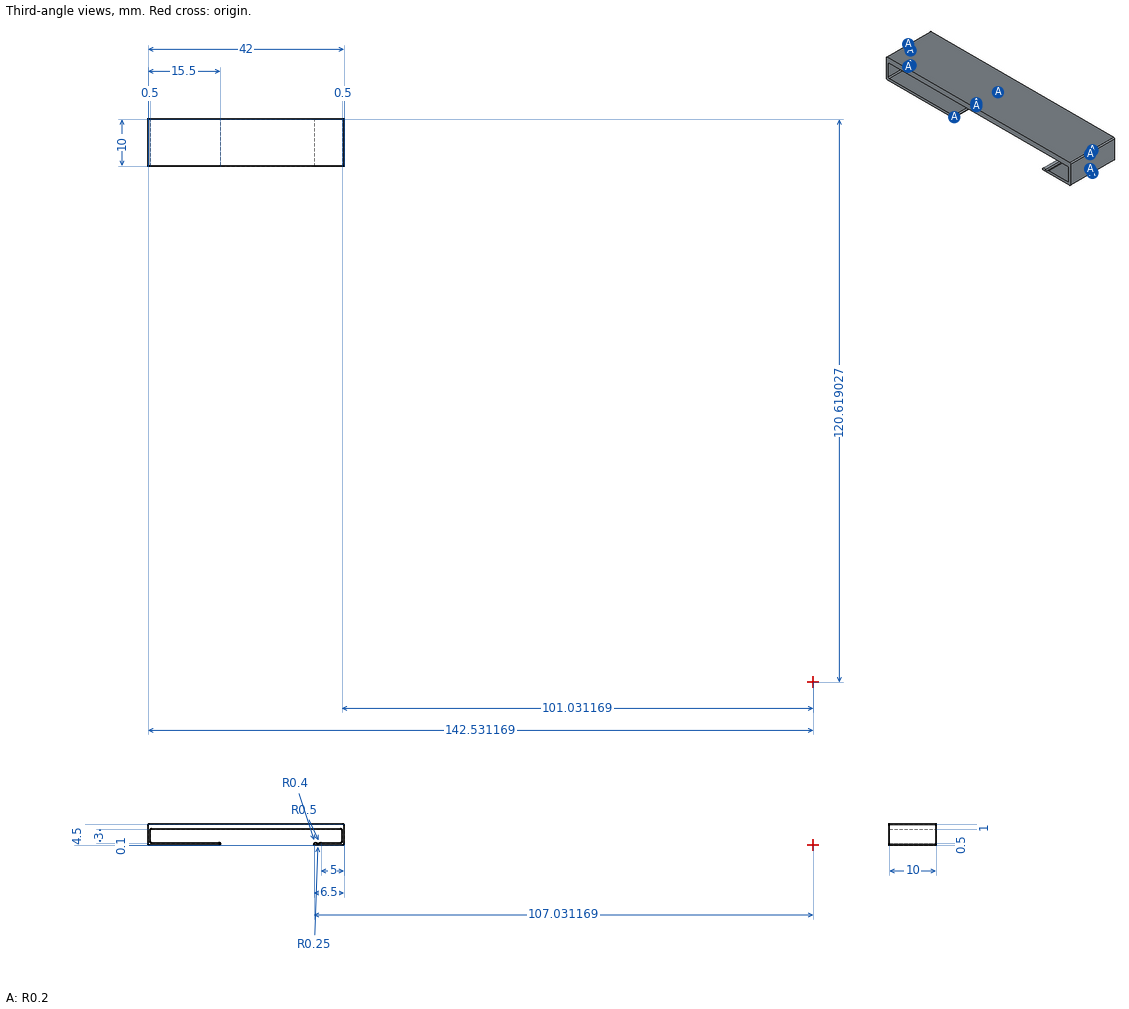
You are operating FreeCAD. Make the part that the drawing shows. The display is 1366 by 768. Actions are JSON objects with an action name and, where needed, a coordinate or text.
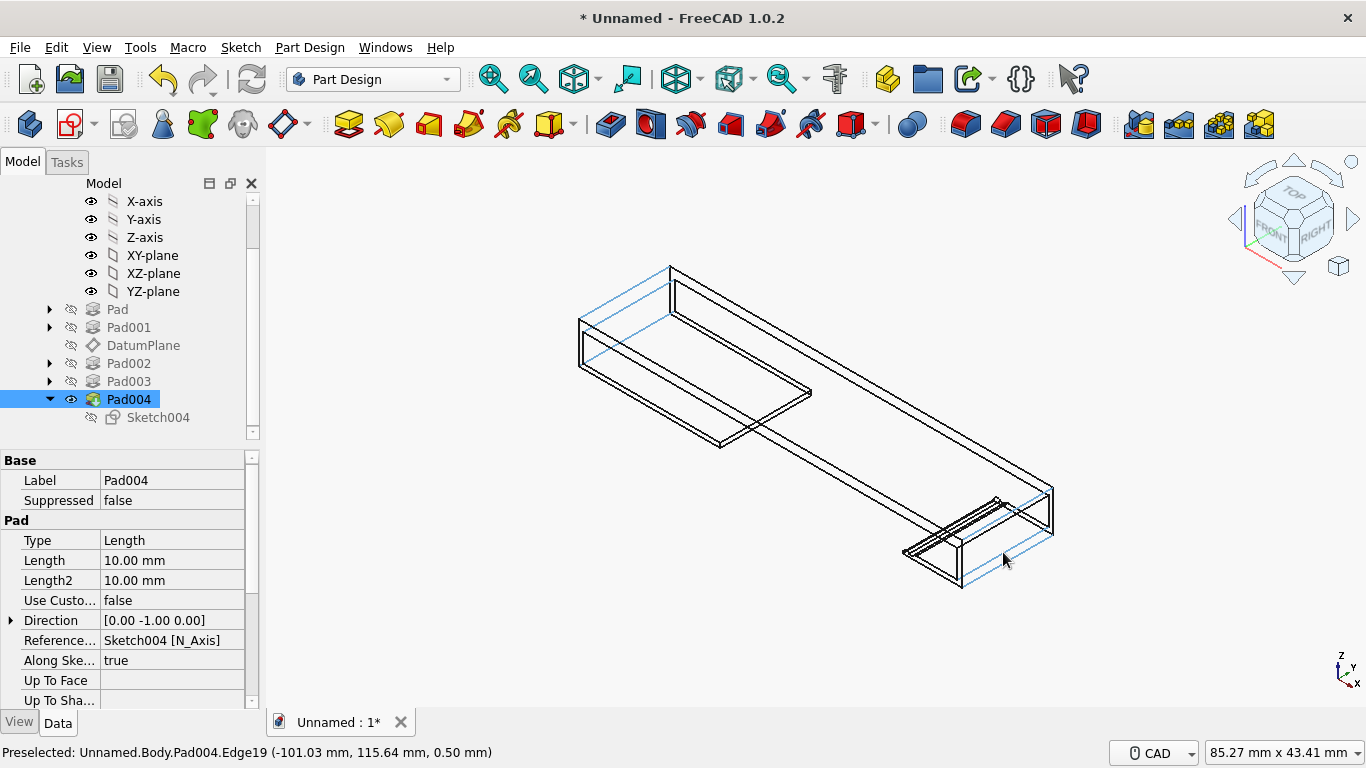
{"action": "scroll", "coordinate": [1003, 521], "scroll_direction": "up", "scroll_amount": 6}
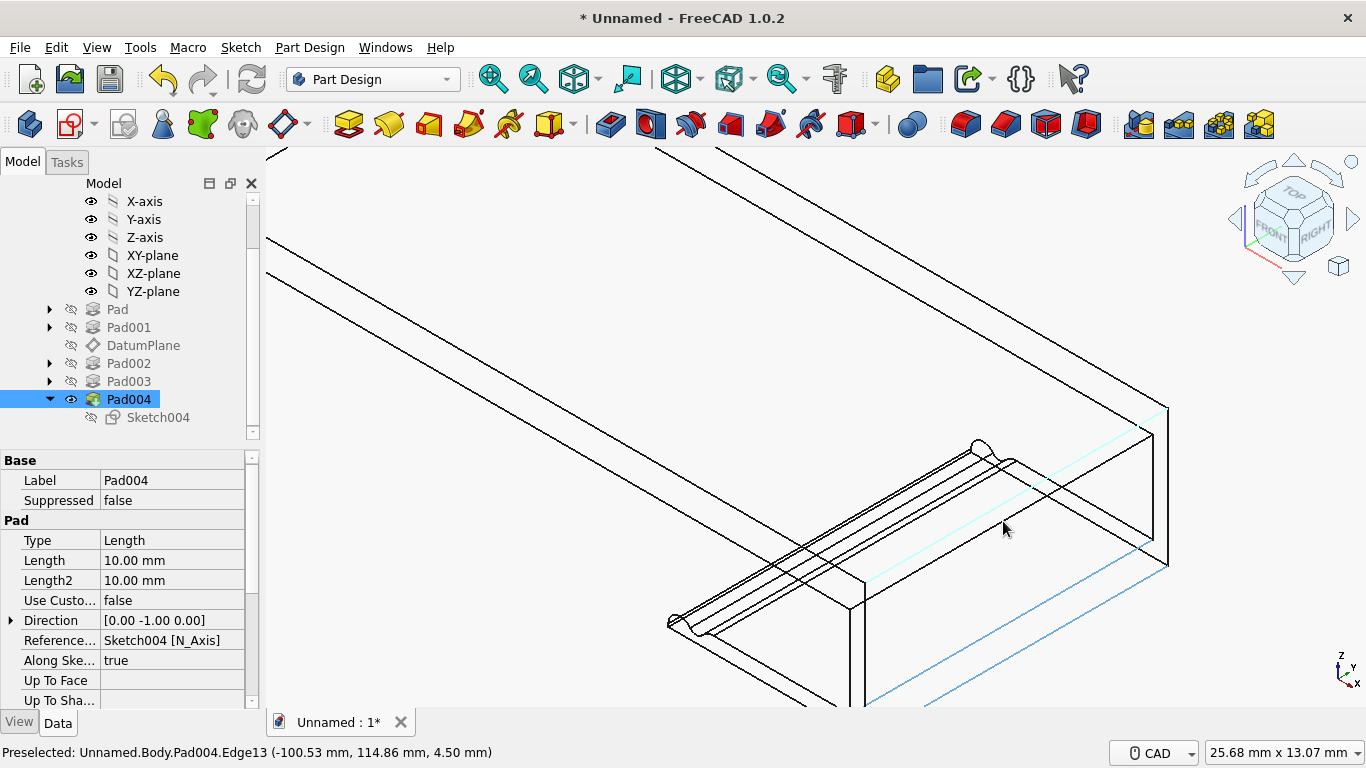
{"action": "left_click", "coordinate": [1001, 521], "text": "ctrl"}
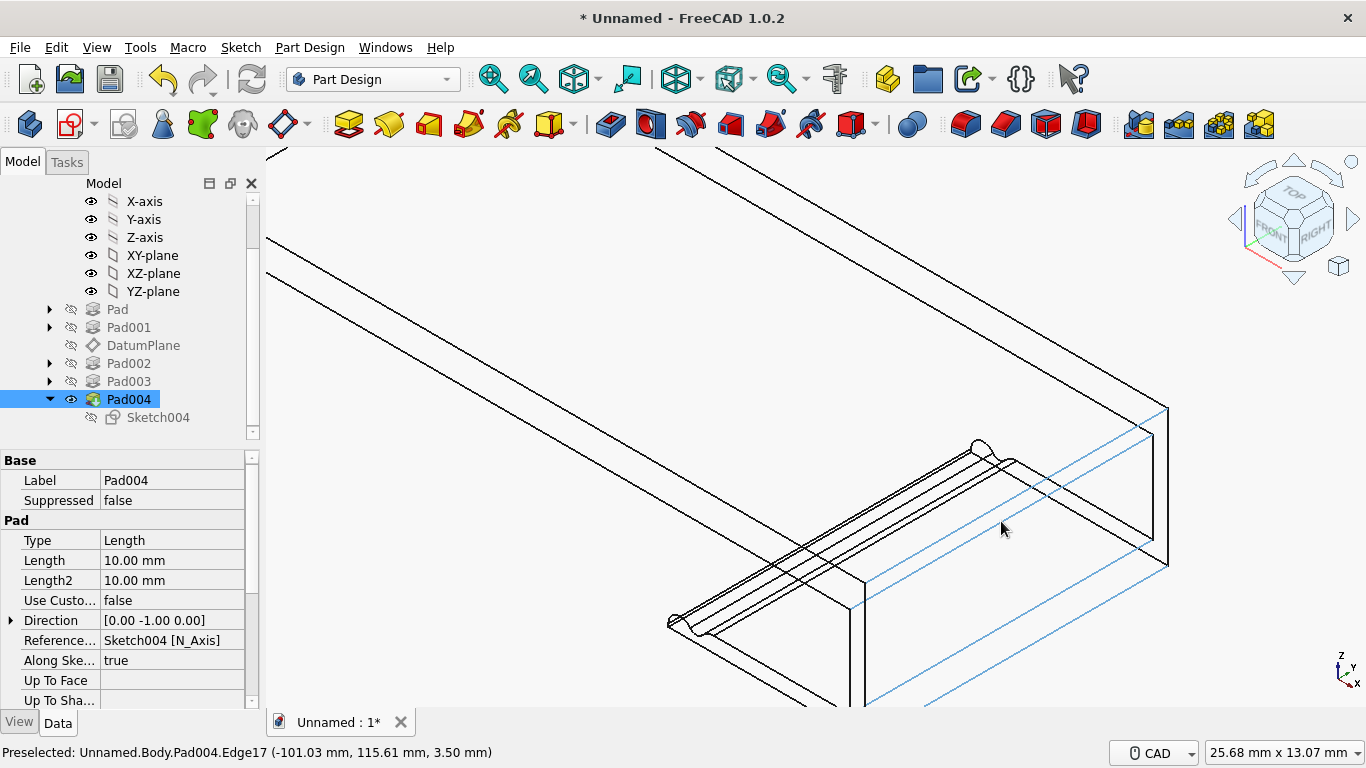
{"action": "key", "text": "v 1"}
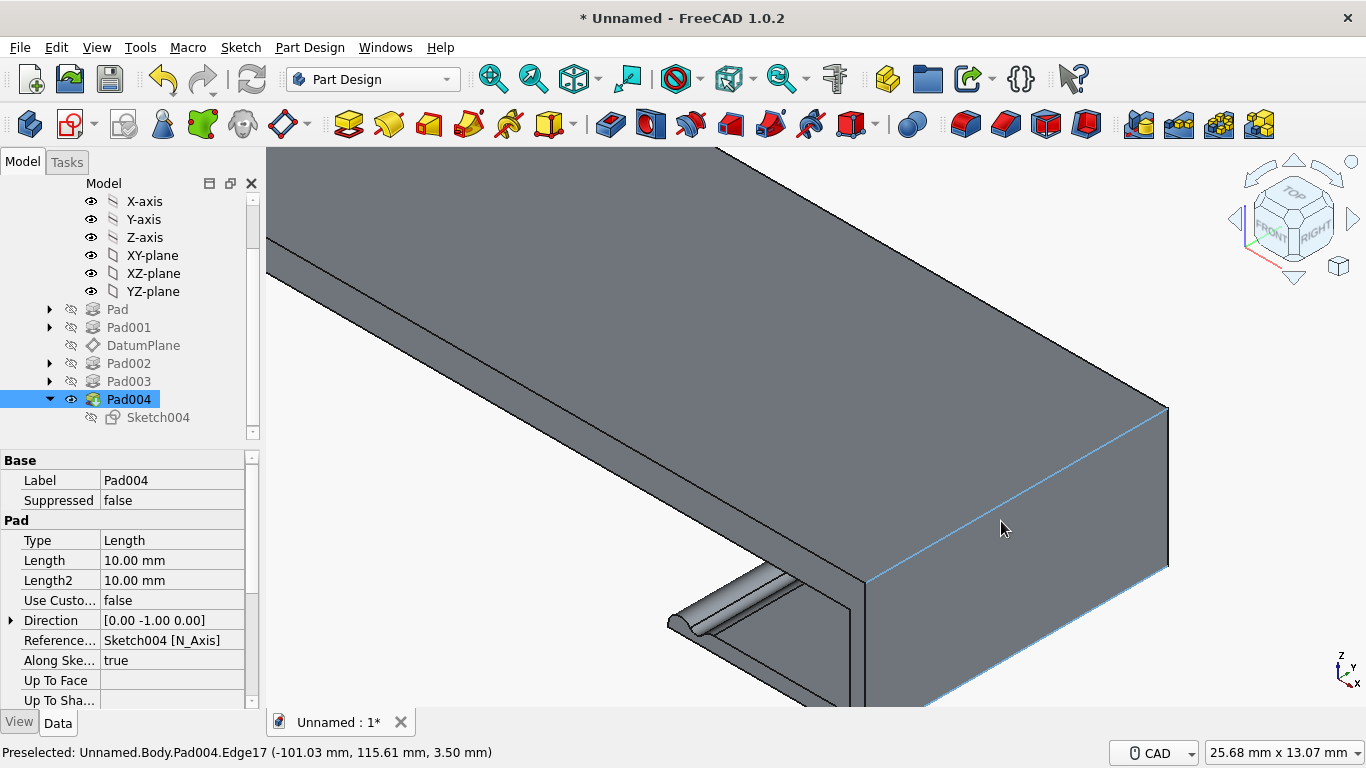
{"action": "left_click", "coordinate": [966, 124]}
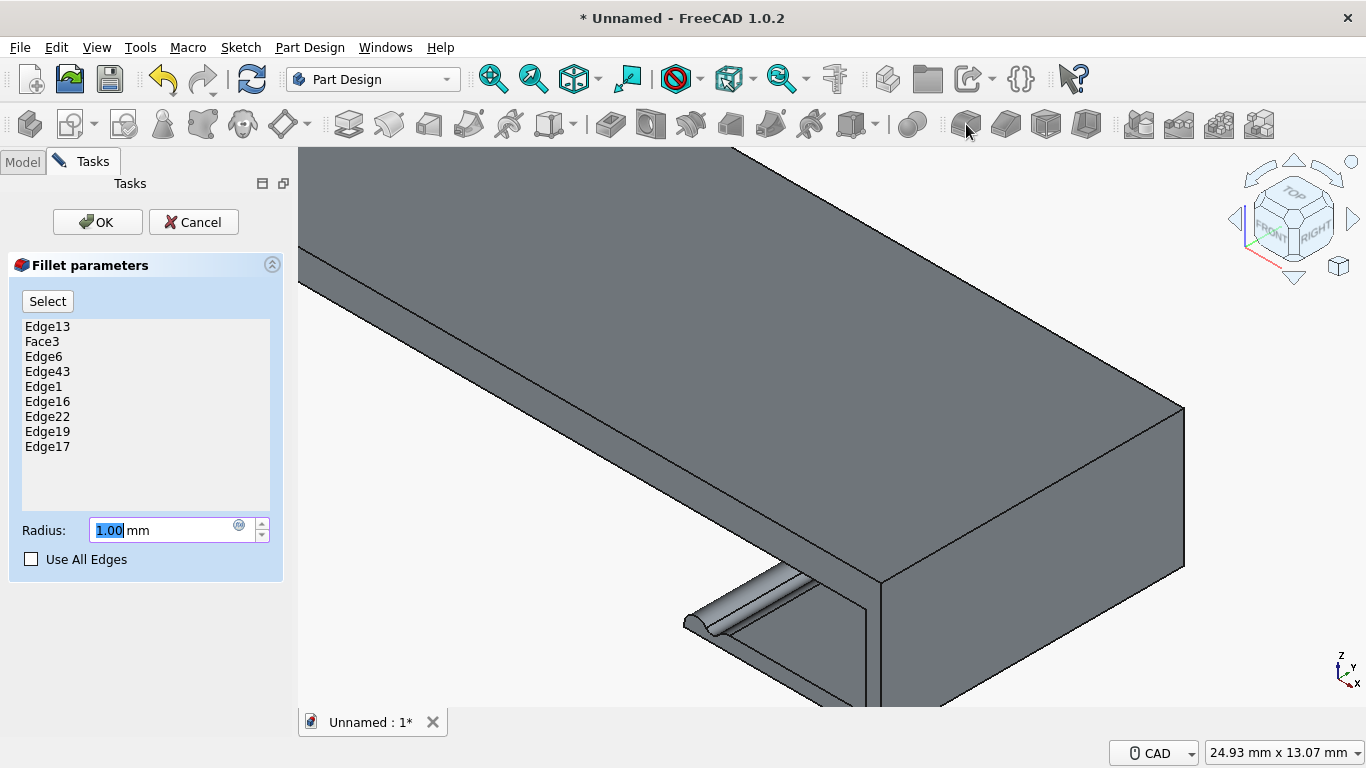
{"action": "type", "text": "0.2"}
{"action": "key", "text": "Tab"}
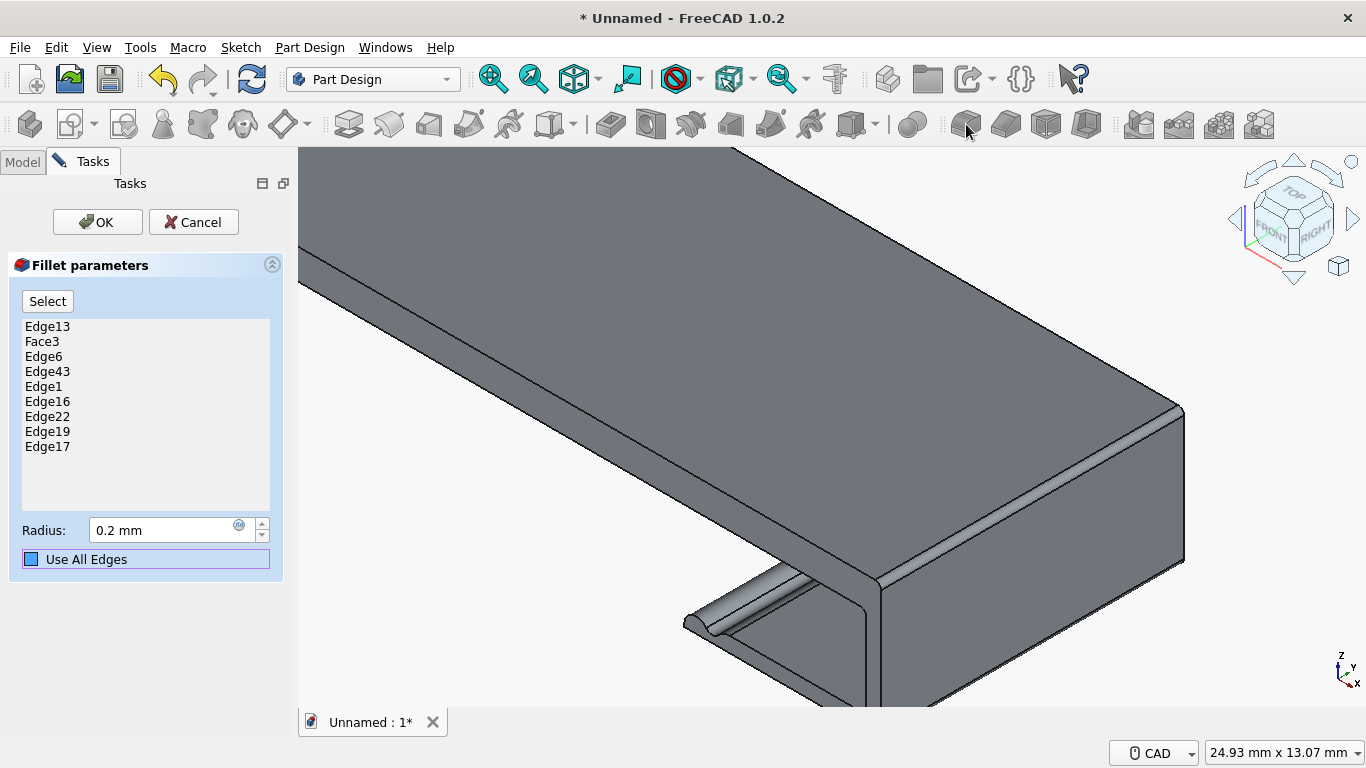
{"action": "left_click", "coordinate": [98, 222]}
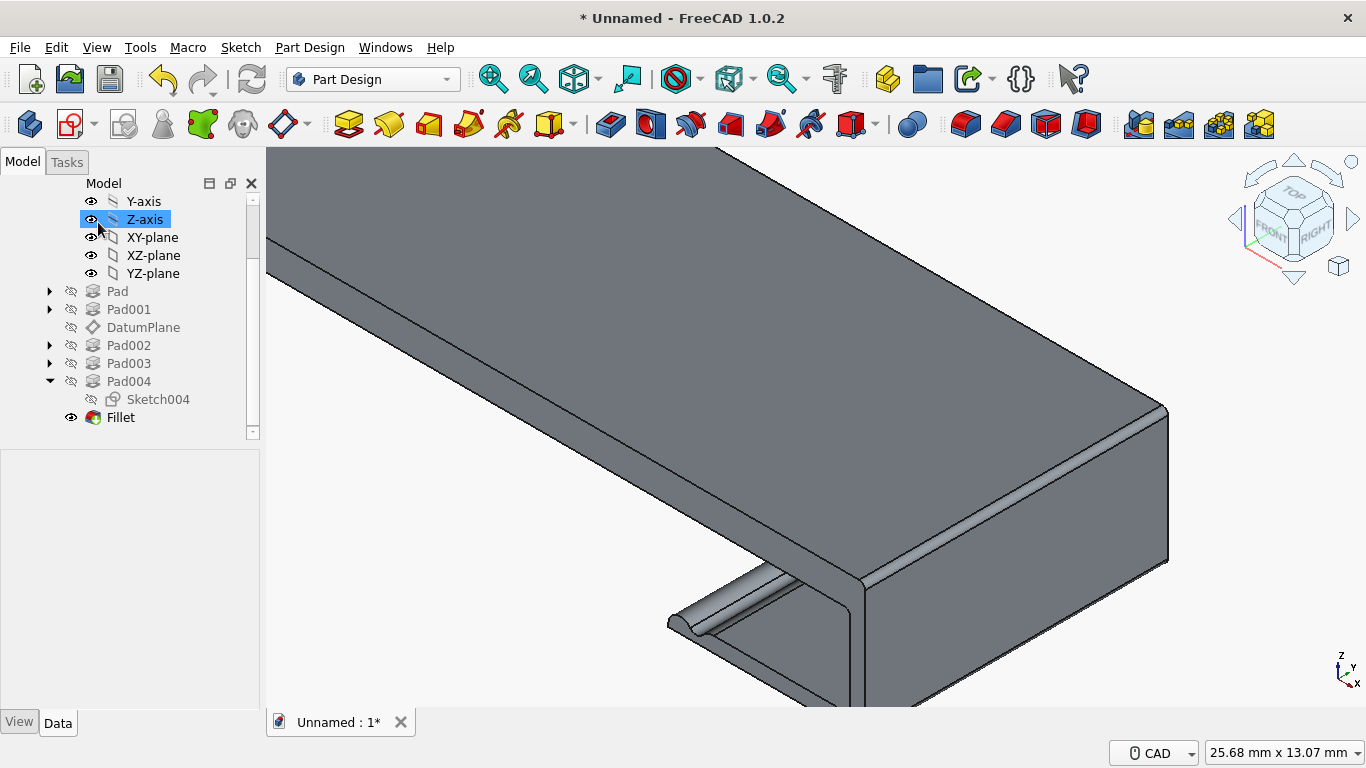
{"action": "left_click", "coordinate": [494, 80]}